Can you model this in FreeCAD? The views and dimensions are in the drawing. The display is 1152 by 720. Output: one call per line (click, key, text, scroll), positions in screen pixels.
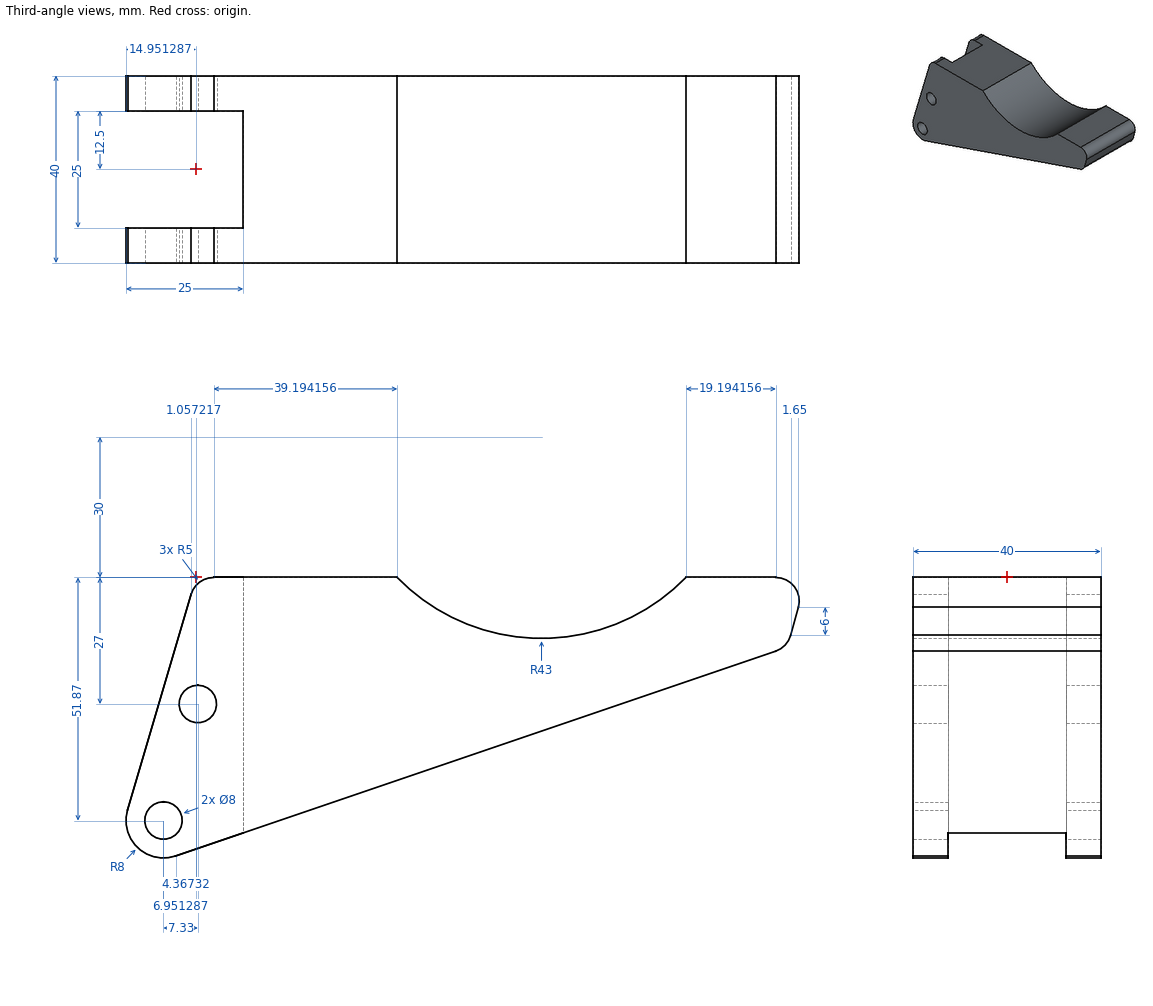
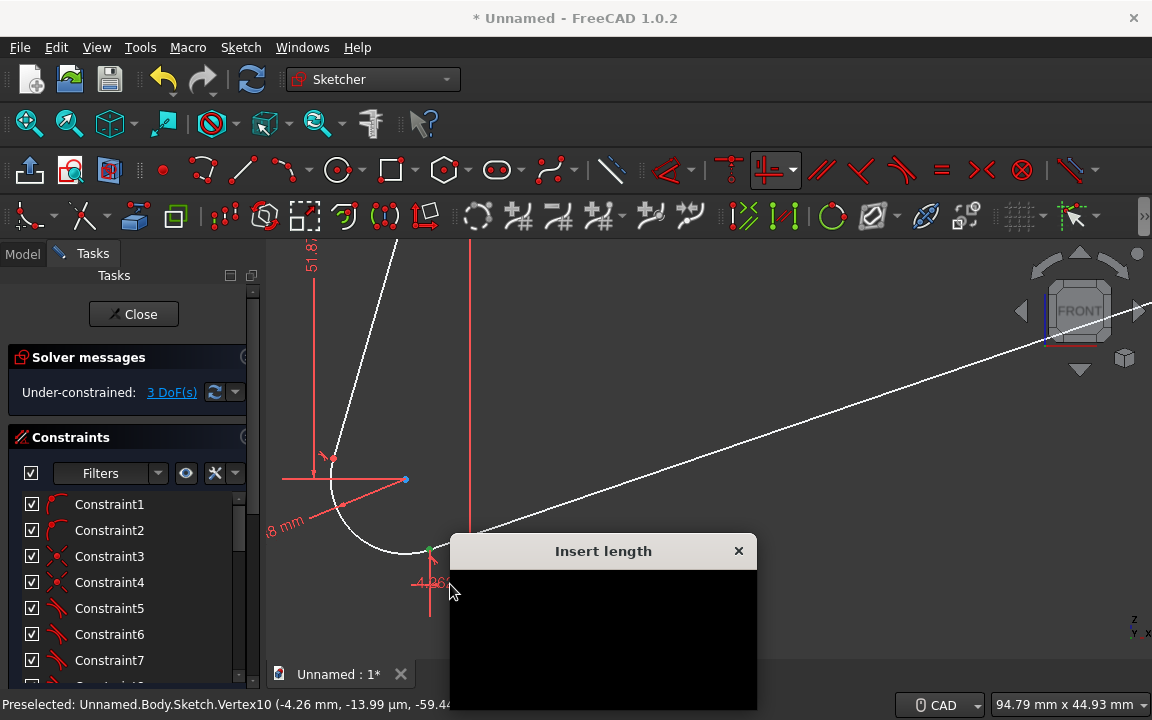
text(4.36732)
key(Return)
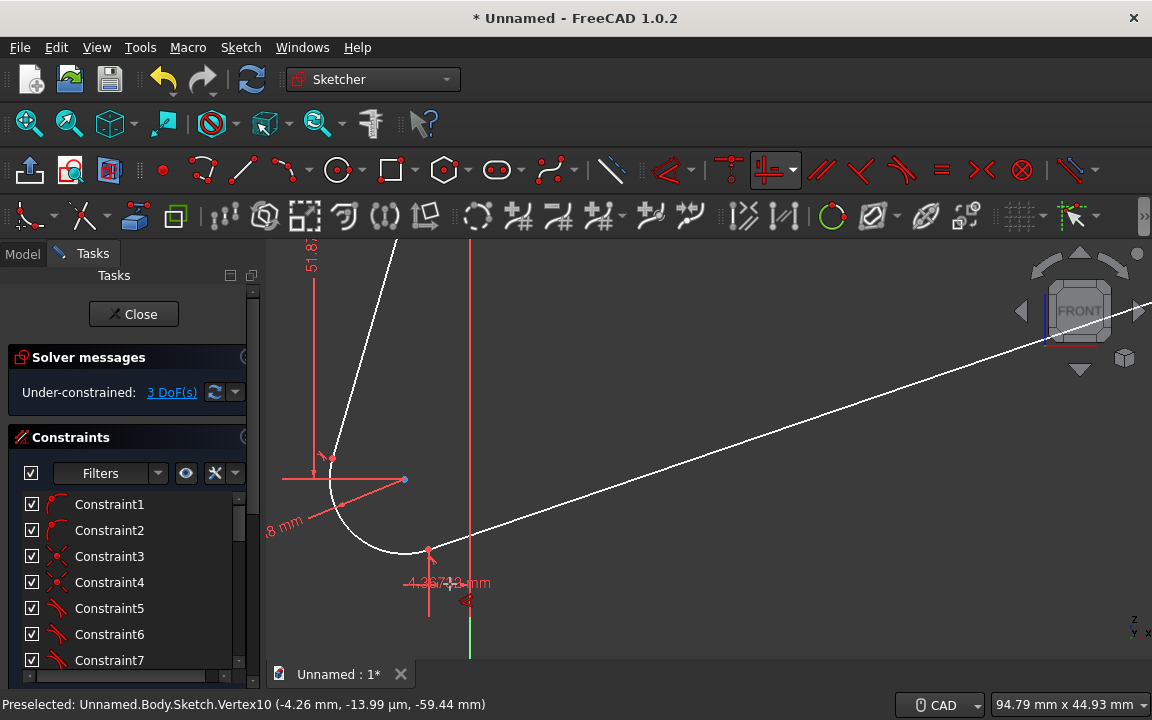
scroll(430, 552, down, 5)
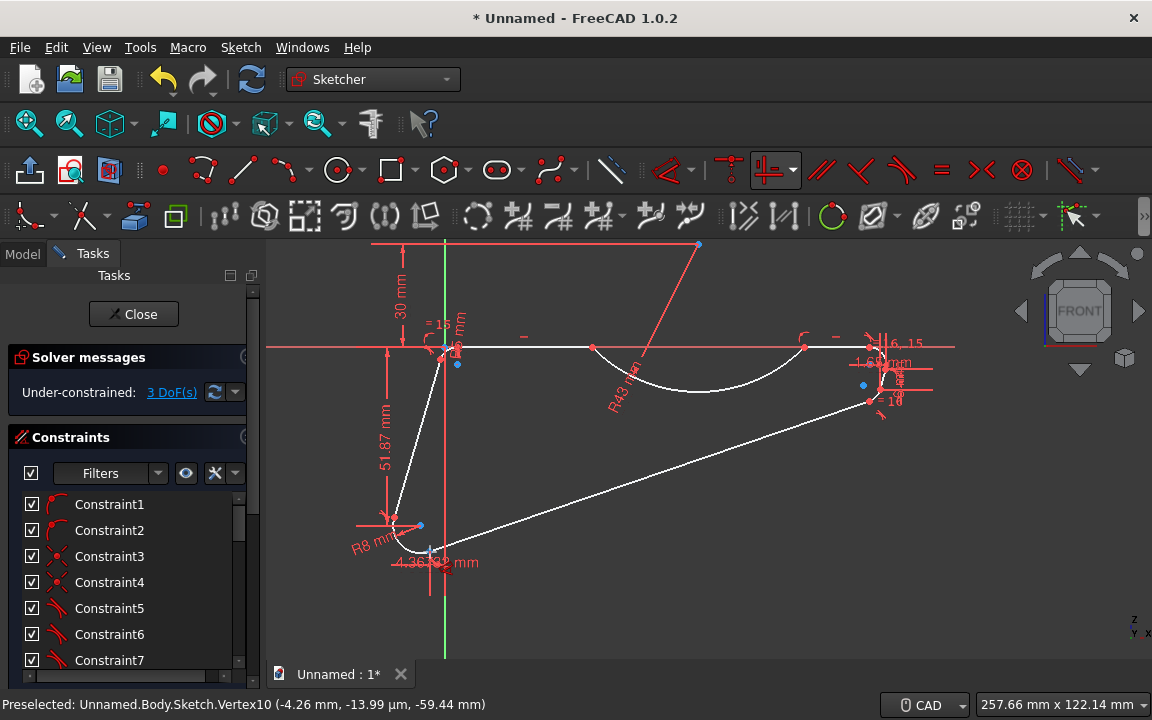
click(498, 347)
click(525, 313)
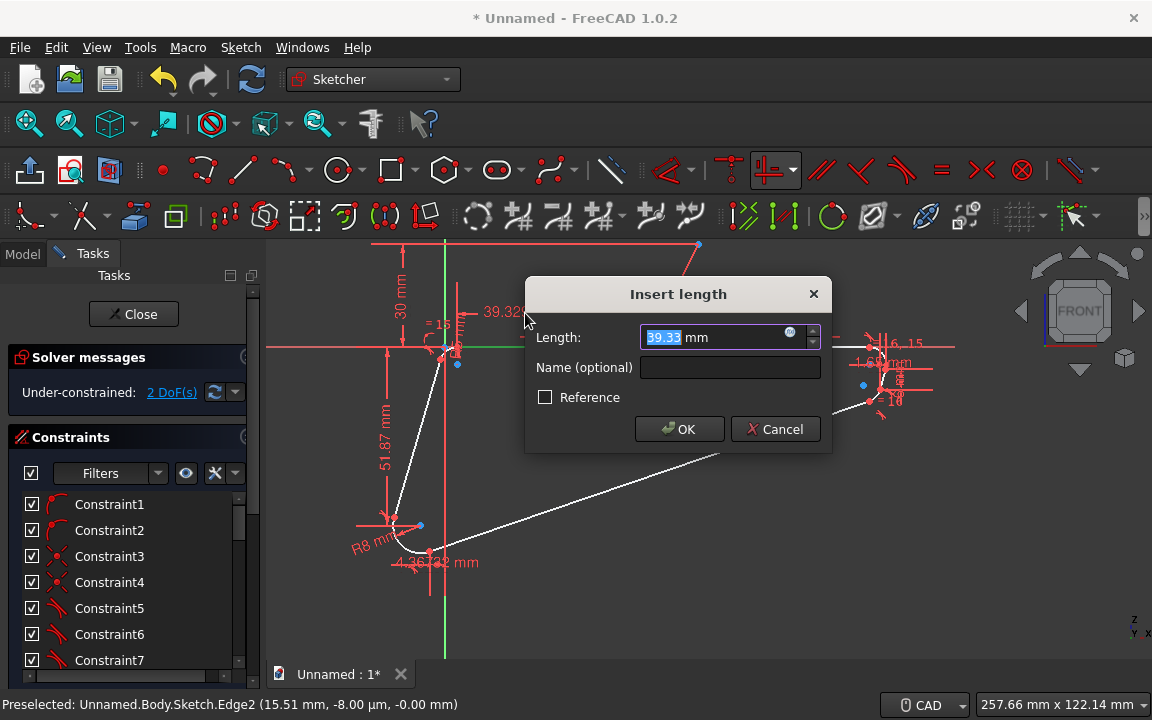
text(39.194156)
key(Return)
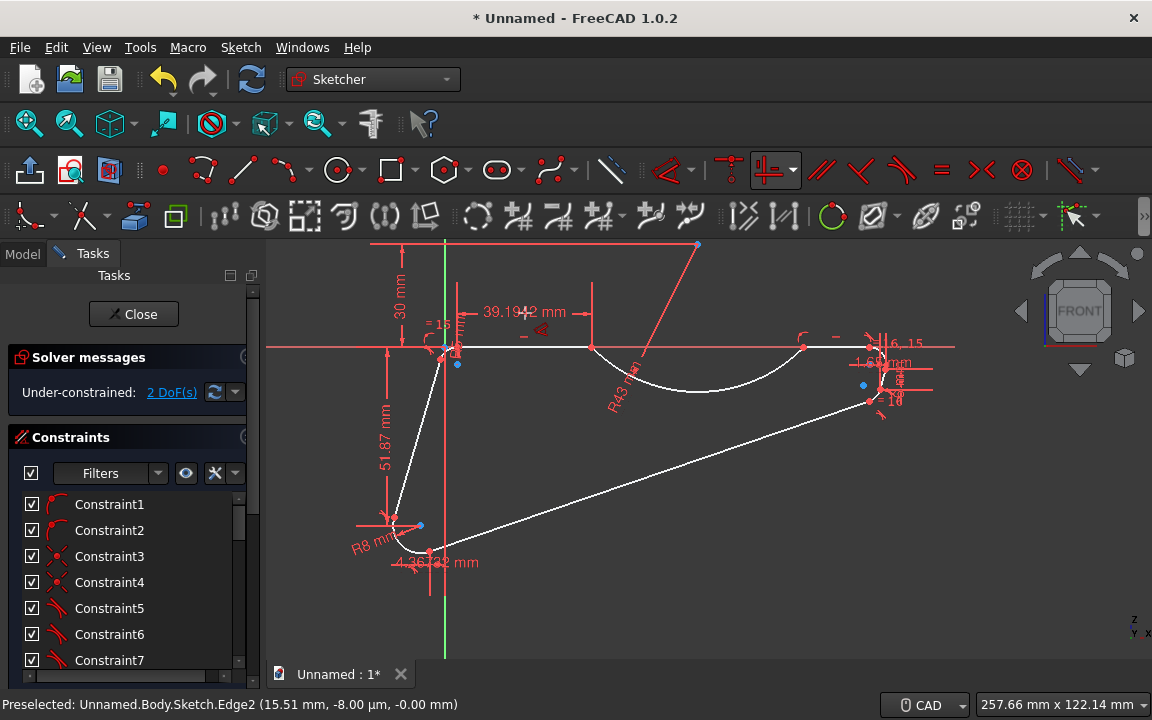
click(823, 347)
click(836, 313)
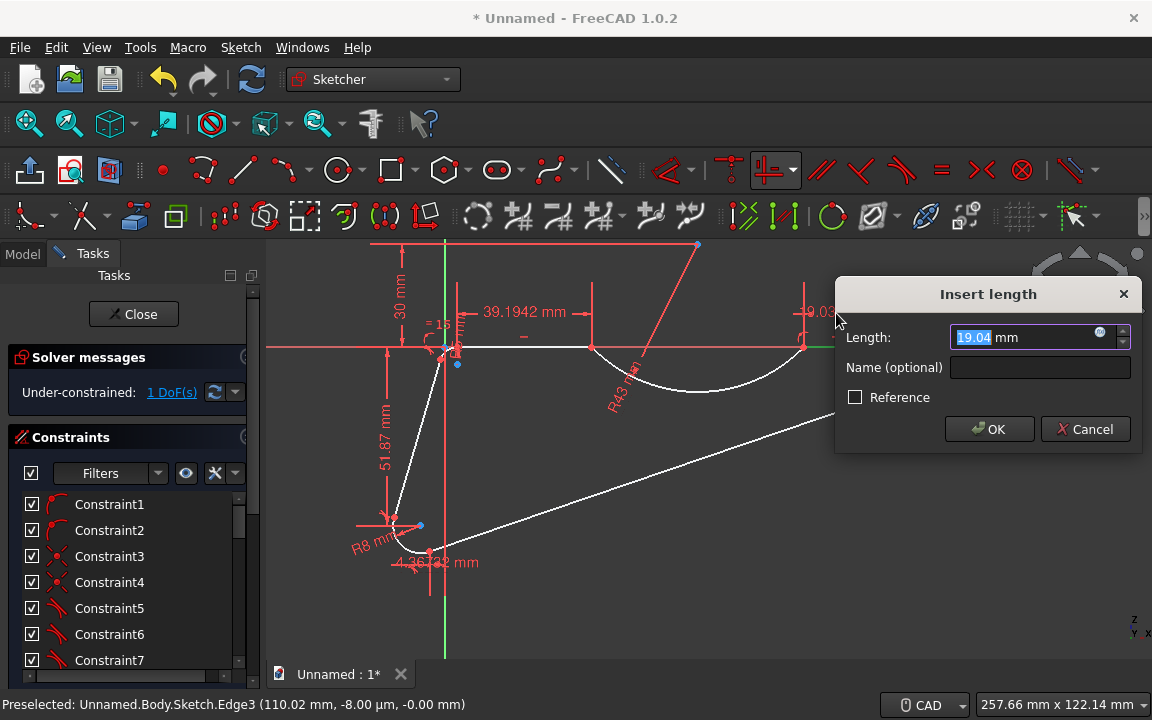
text(19.194156)
key(Return)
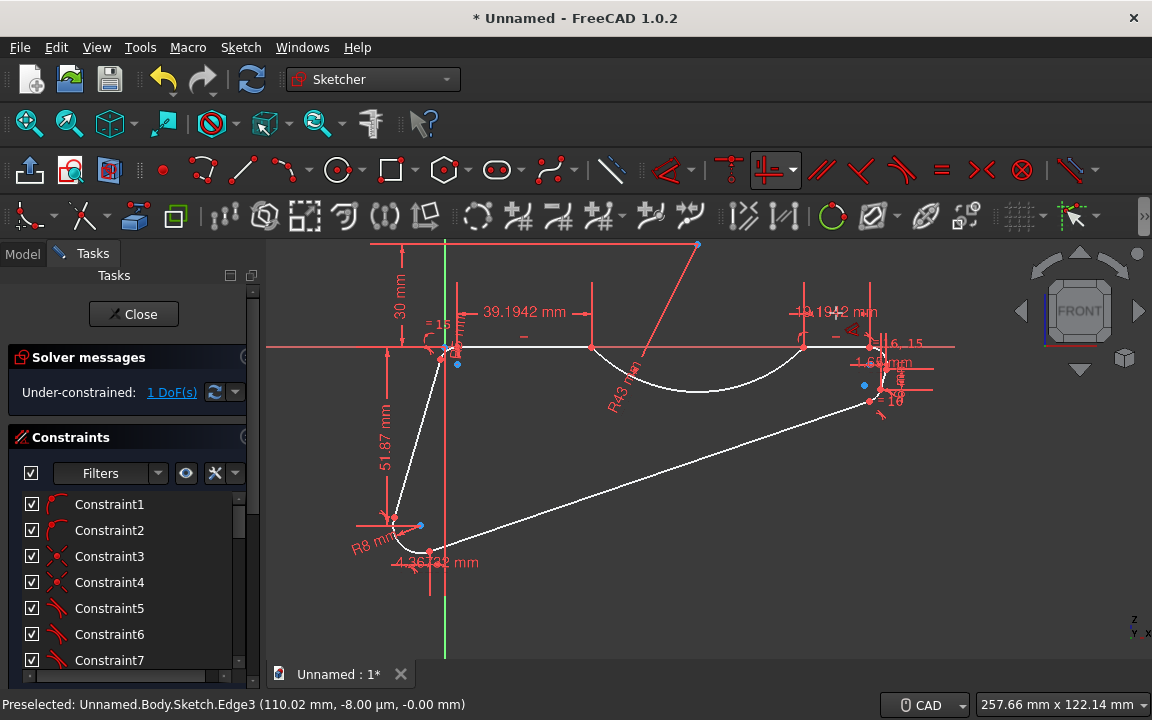
scroll(441, 360, up, 12)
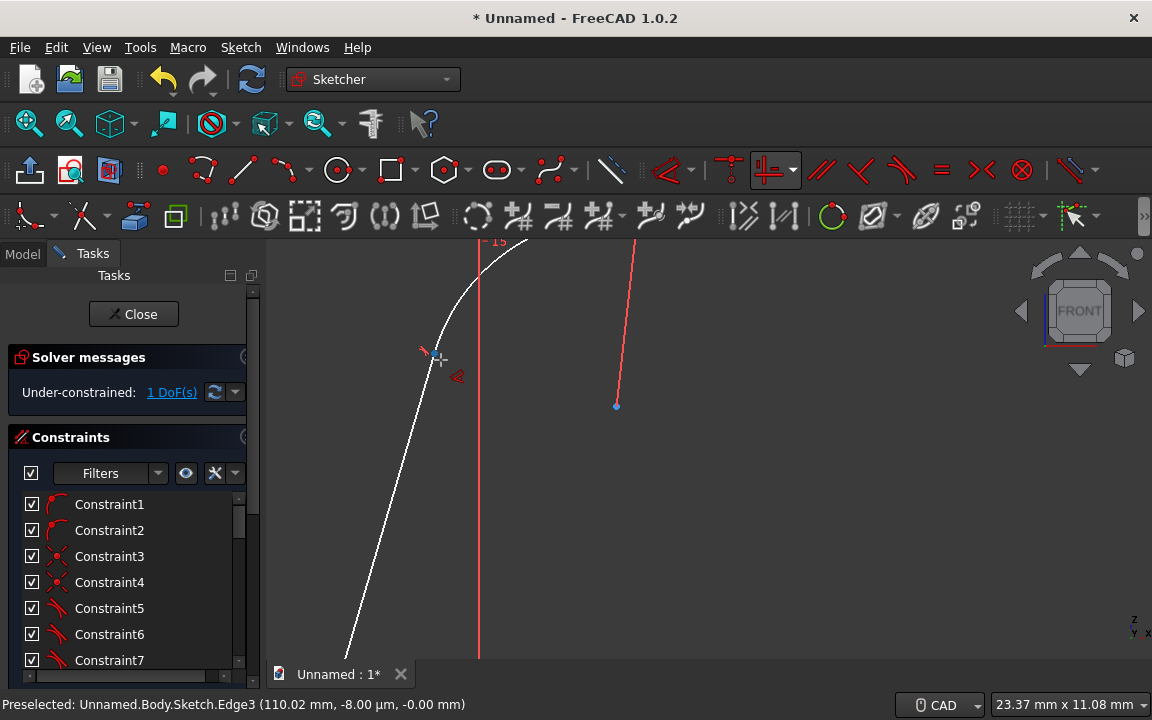
click(435, 353)
click(457, 387)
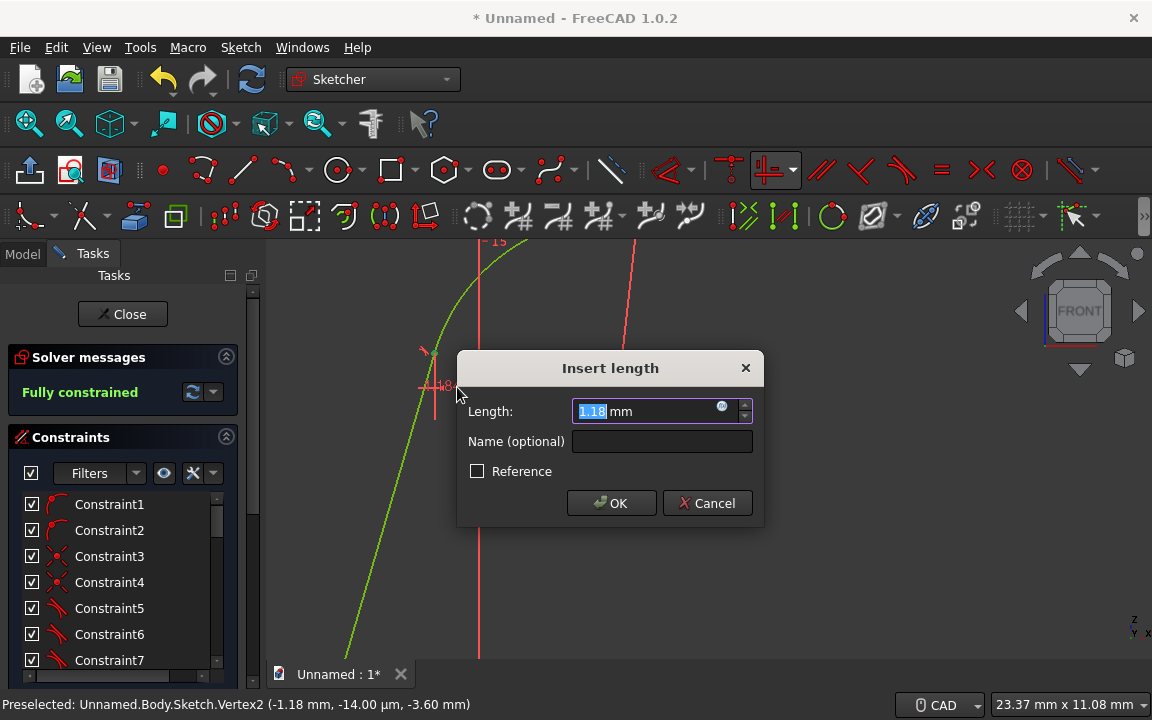
text(1.057217)
key(Return)
key(Escape)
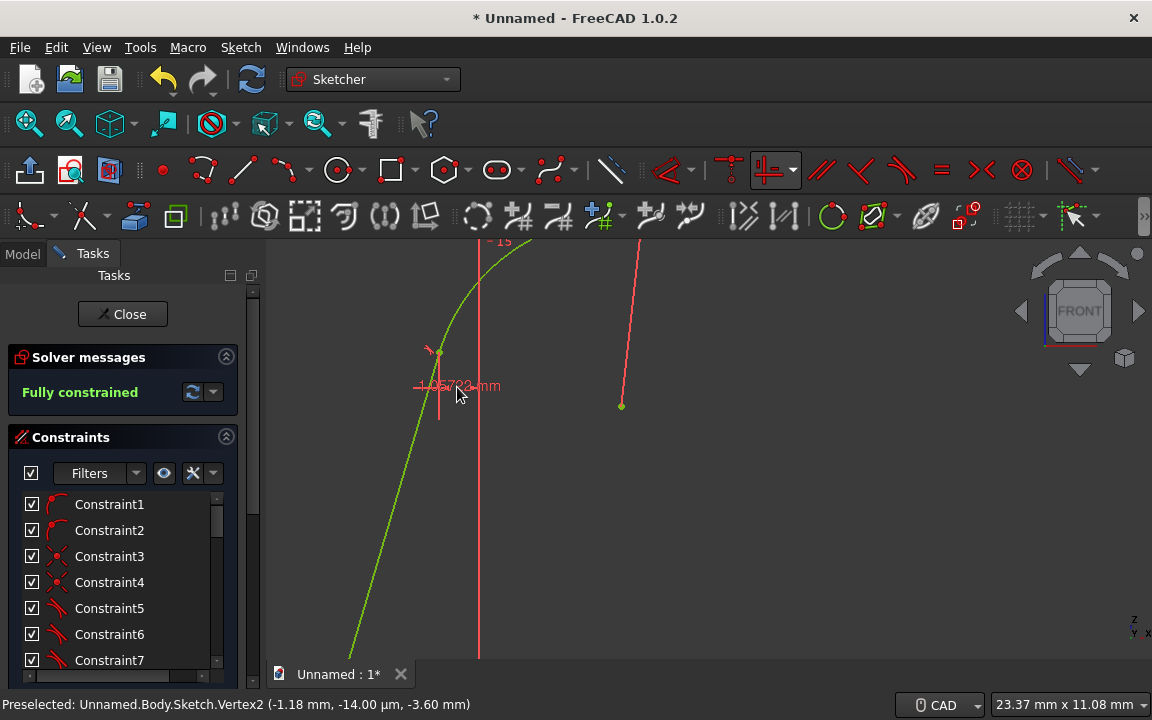
click(123, 314)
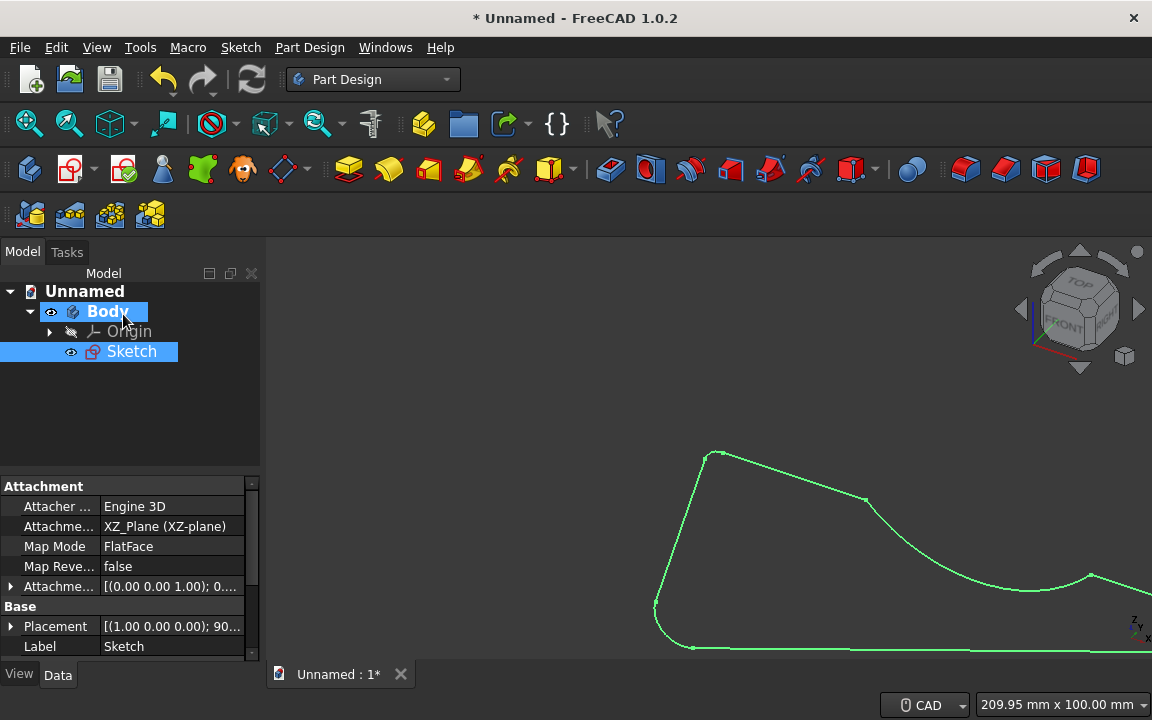
click(350, 170)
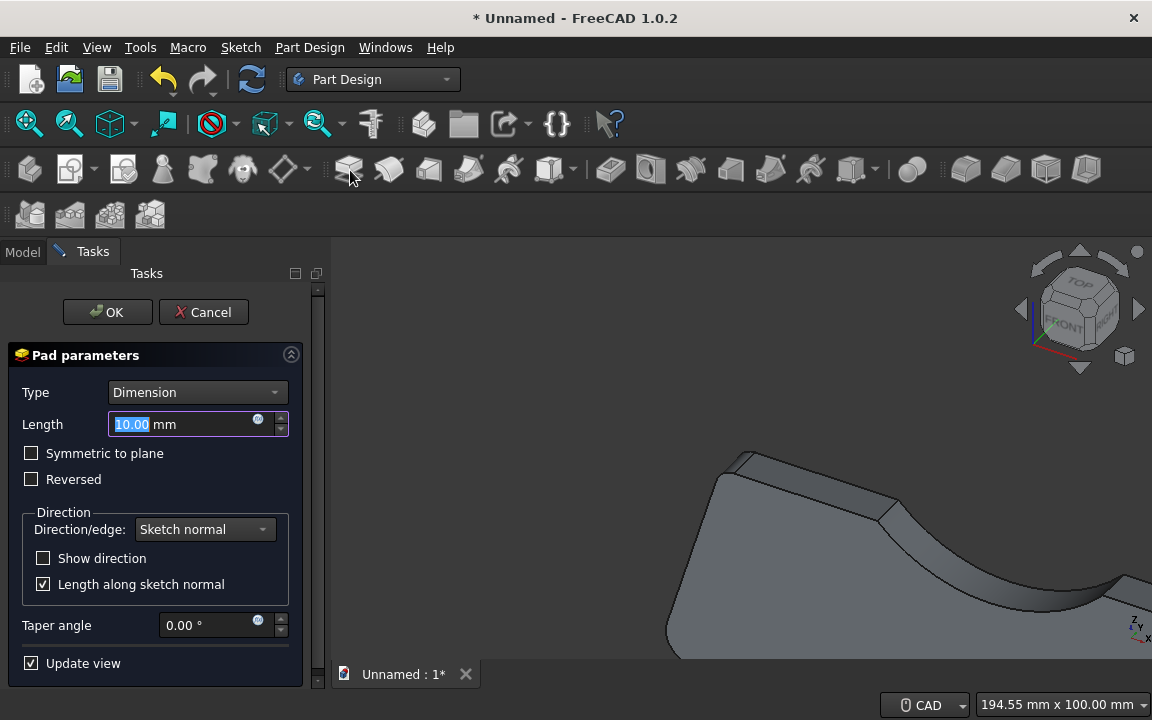
text(40)
key(Tab)